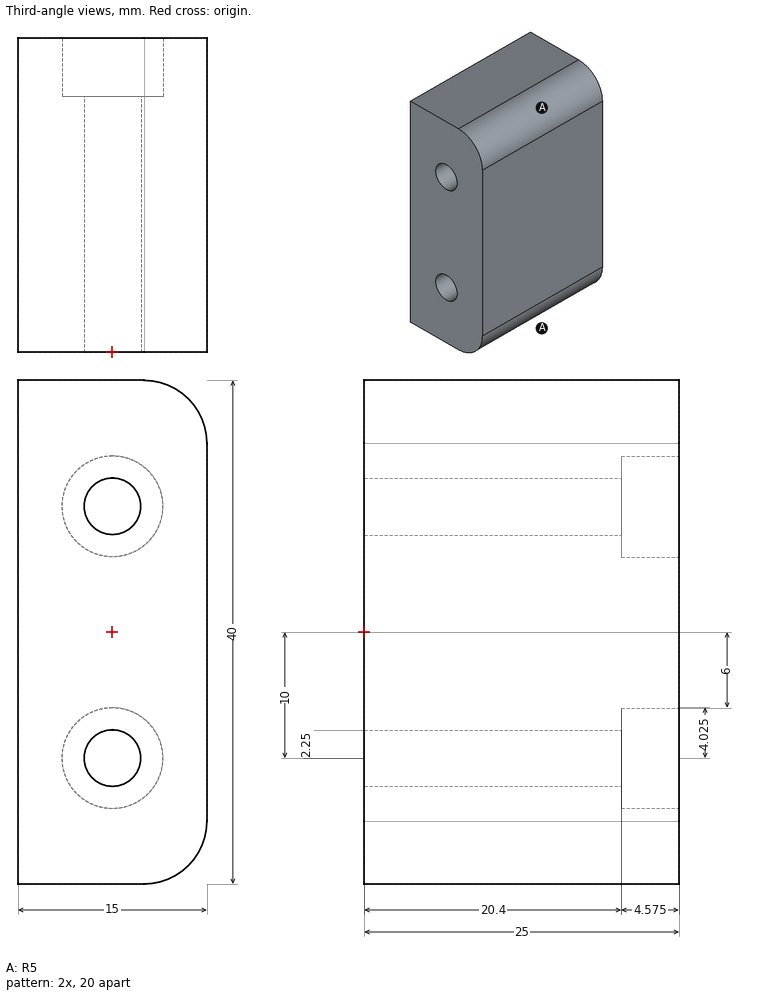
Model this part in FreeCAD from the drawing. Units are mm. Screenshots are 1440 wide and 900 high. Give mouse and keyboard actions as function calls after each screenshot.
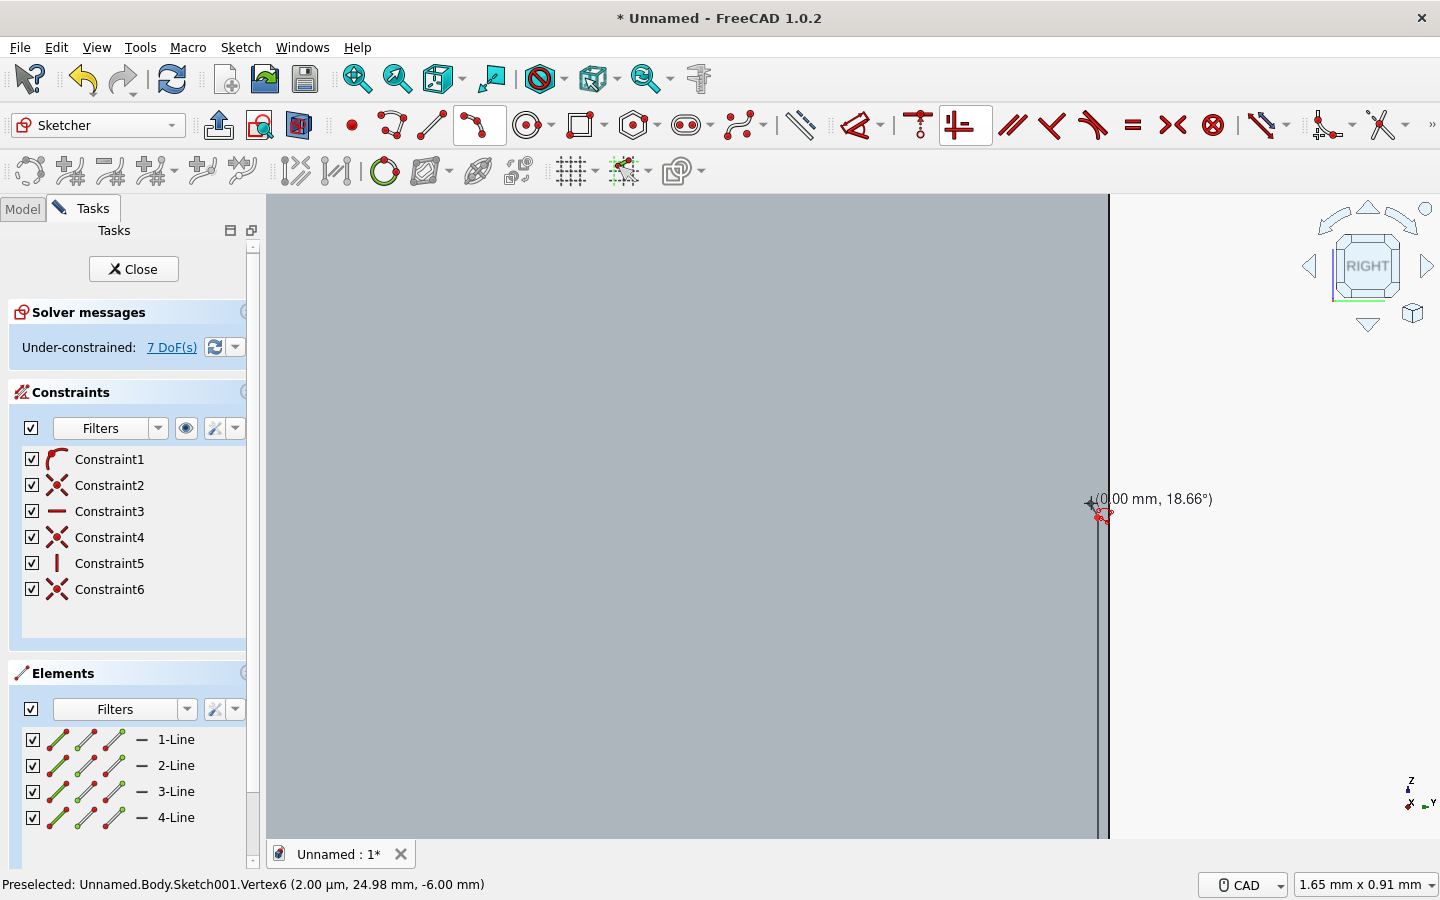
scroll(1203, 542, down, 17)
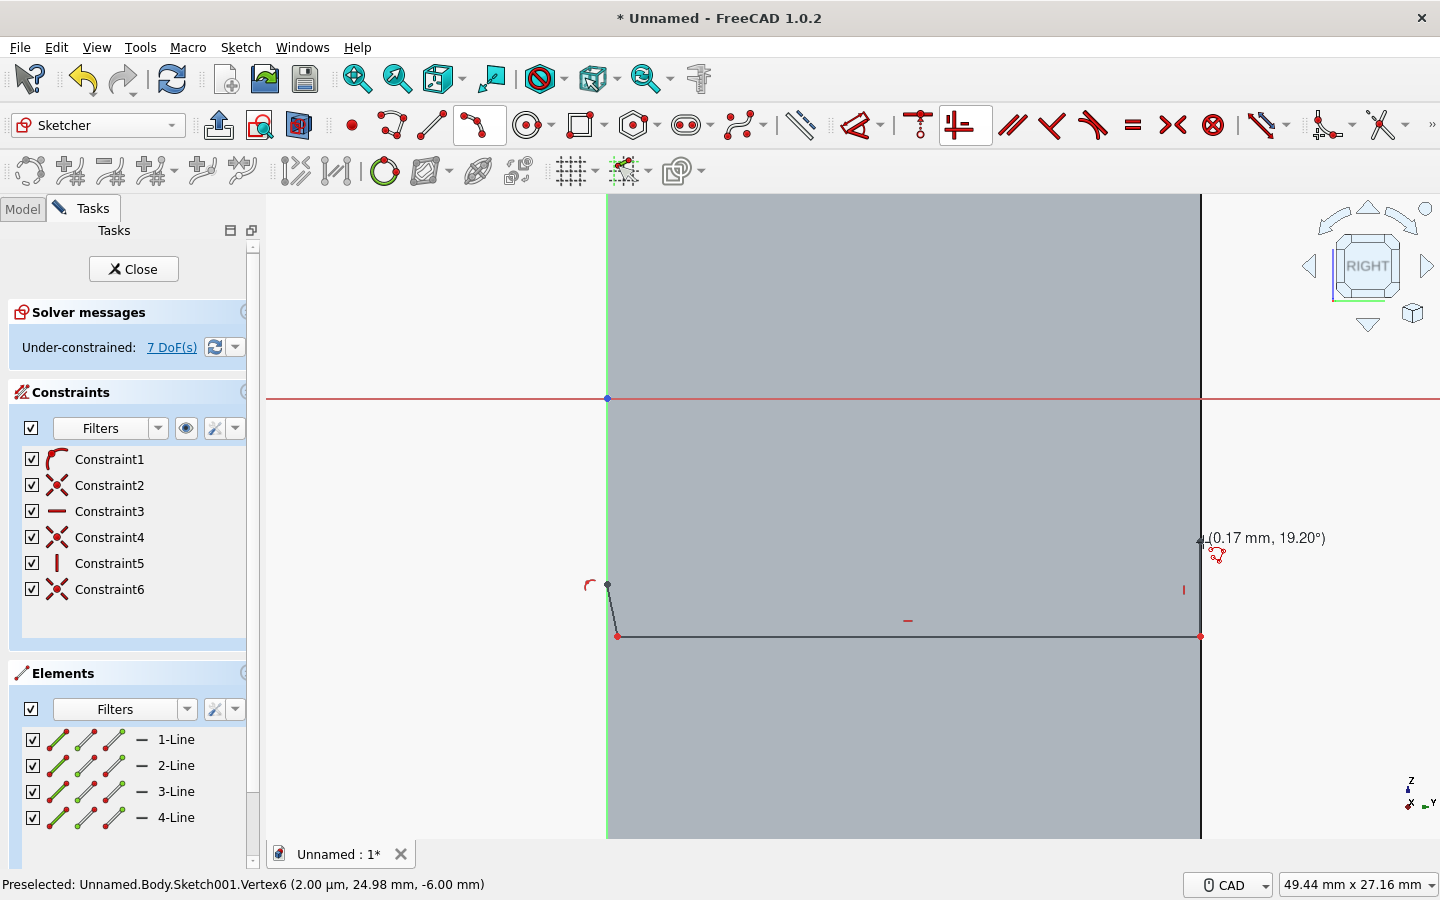
click(1091, 541)
click(1091, 583)
click(607, 584)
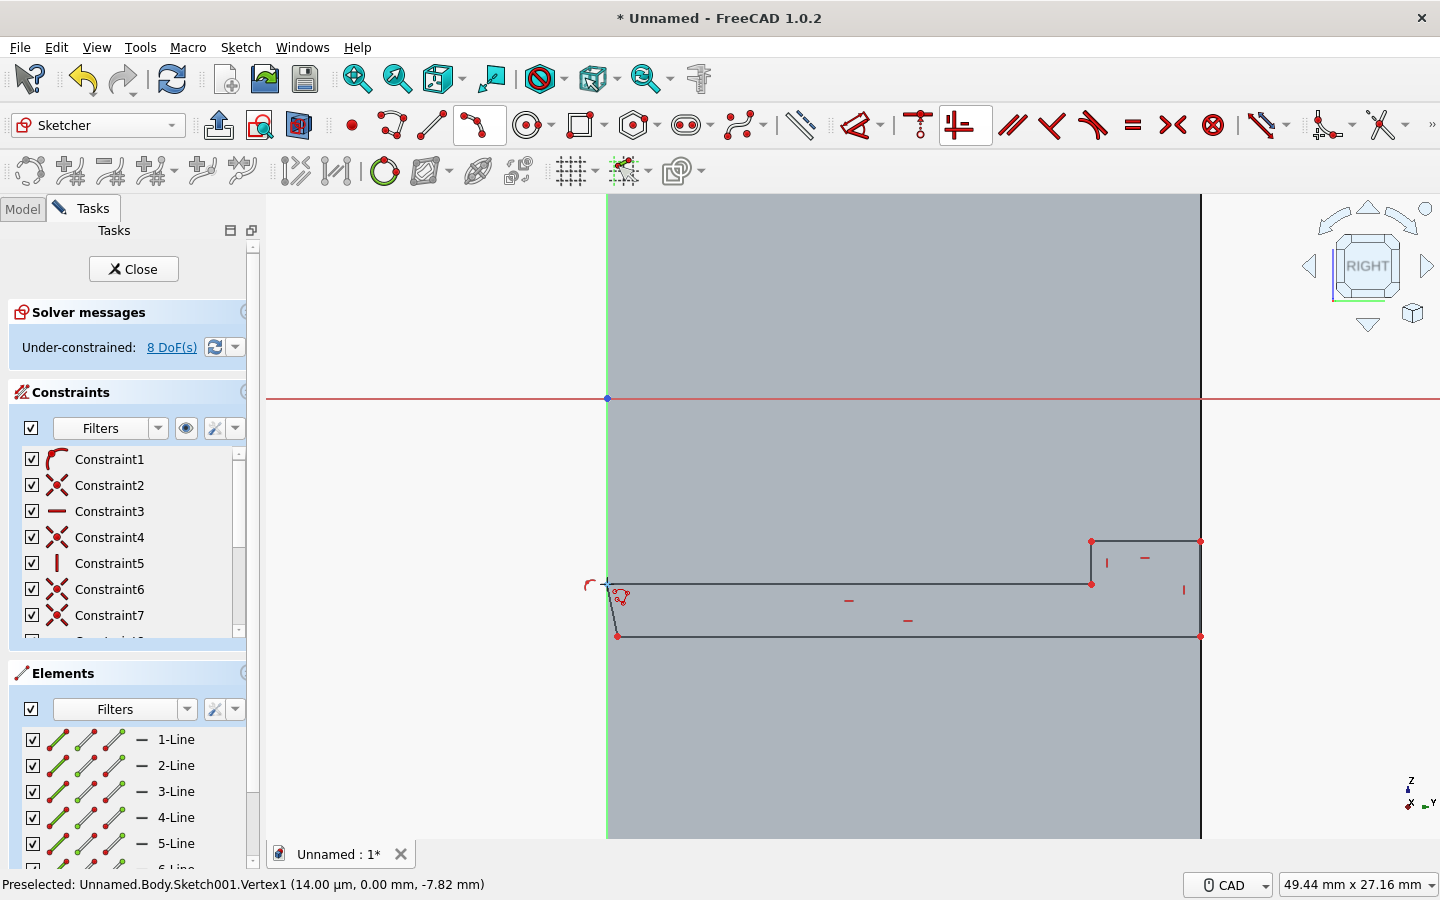
click(432, 126)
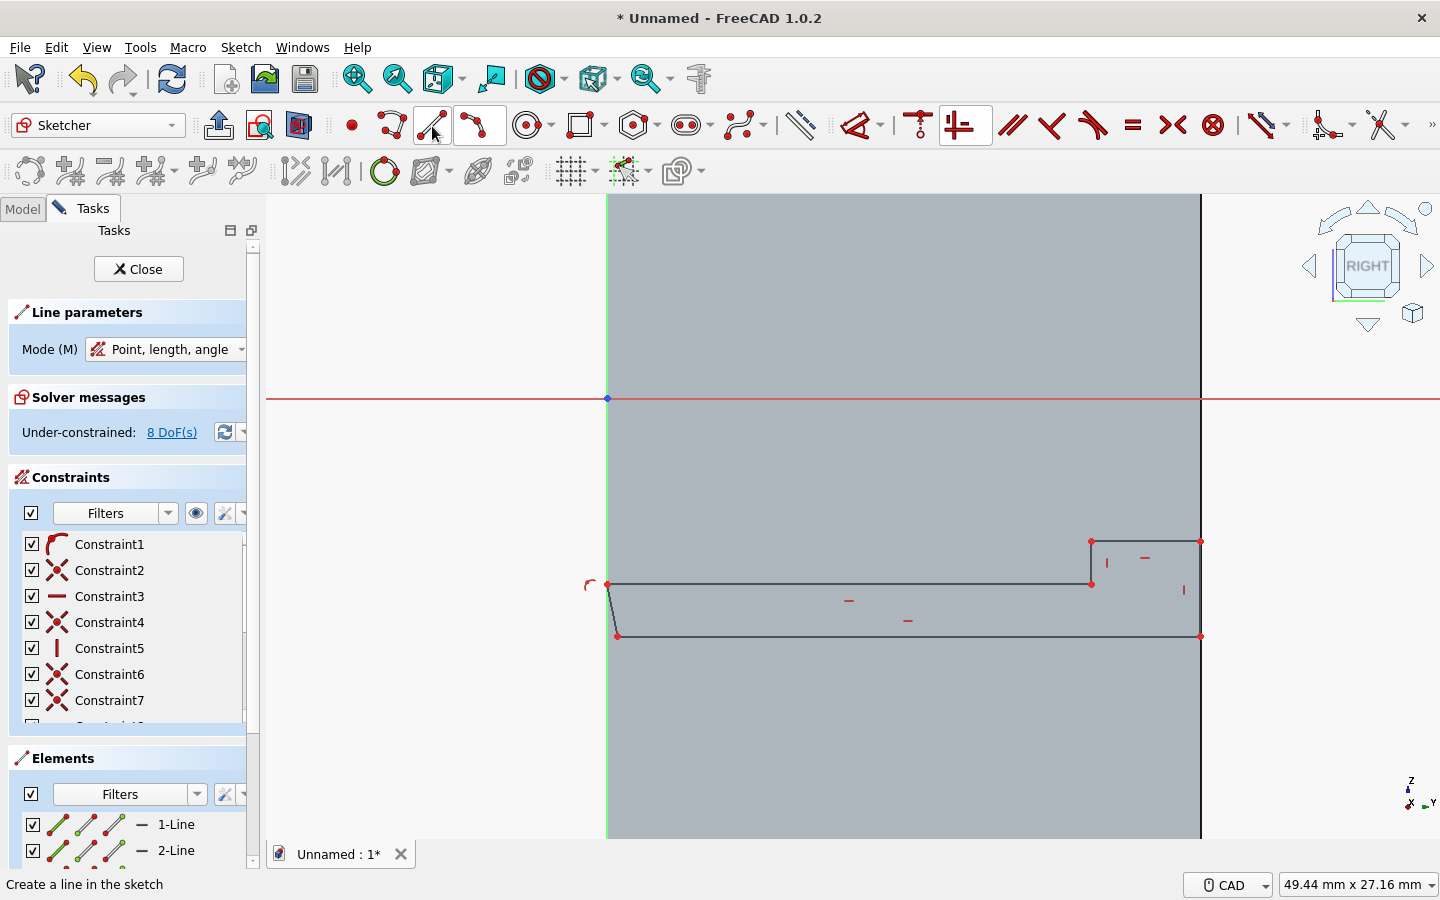
click(548, 636)
click(370, 636)
key(Escape)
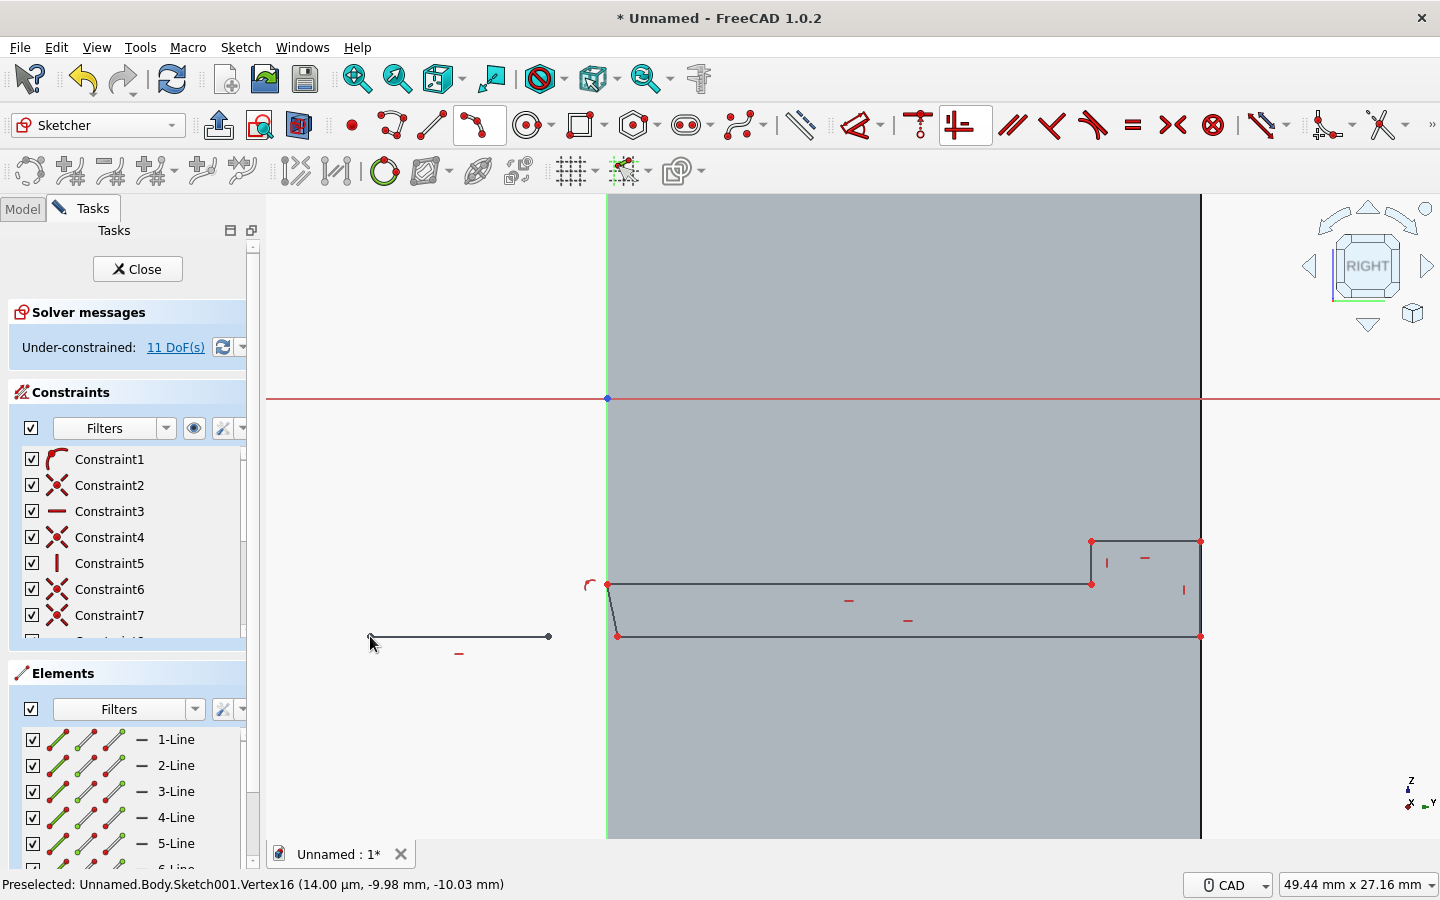
click(495, 637)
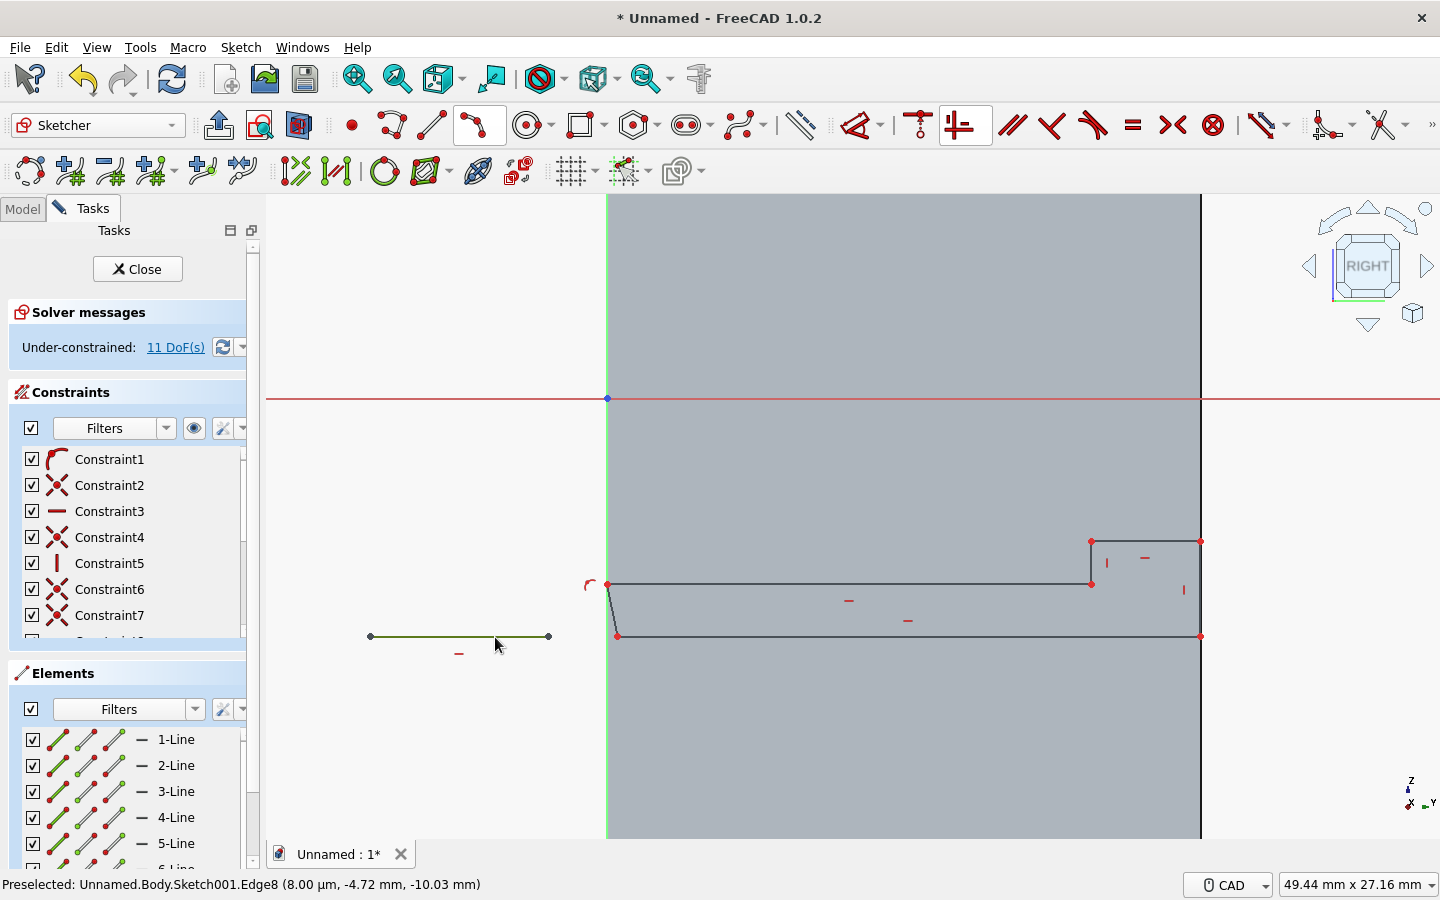
click(802, 126)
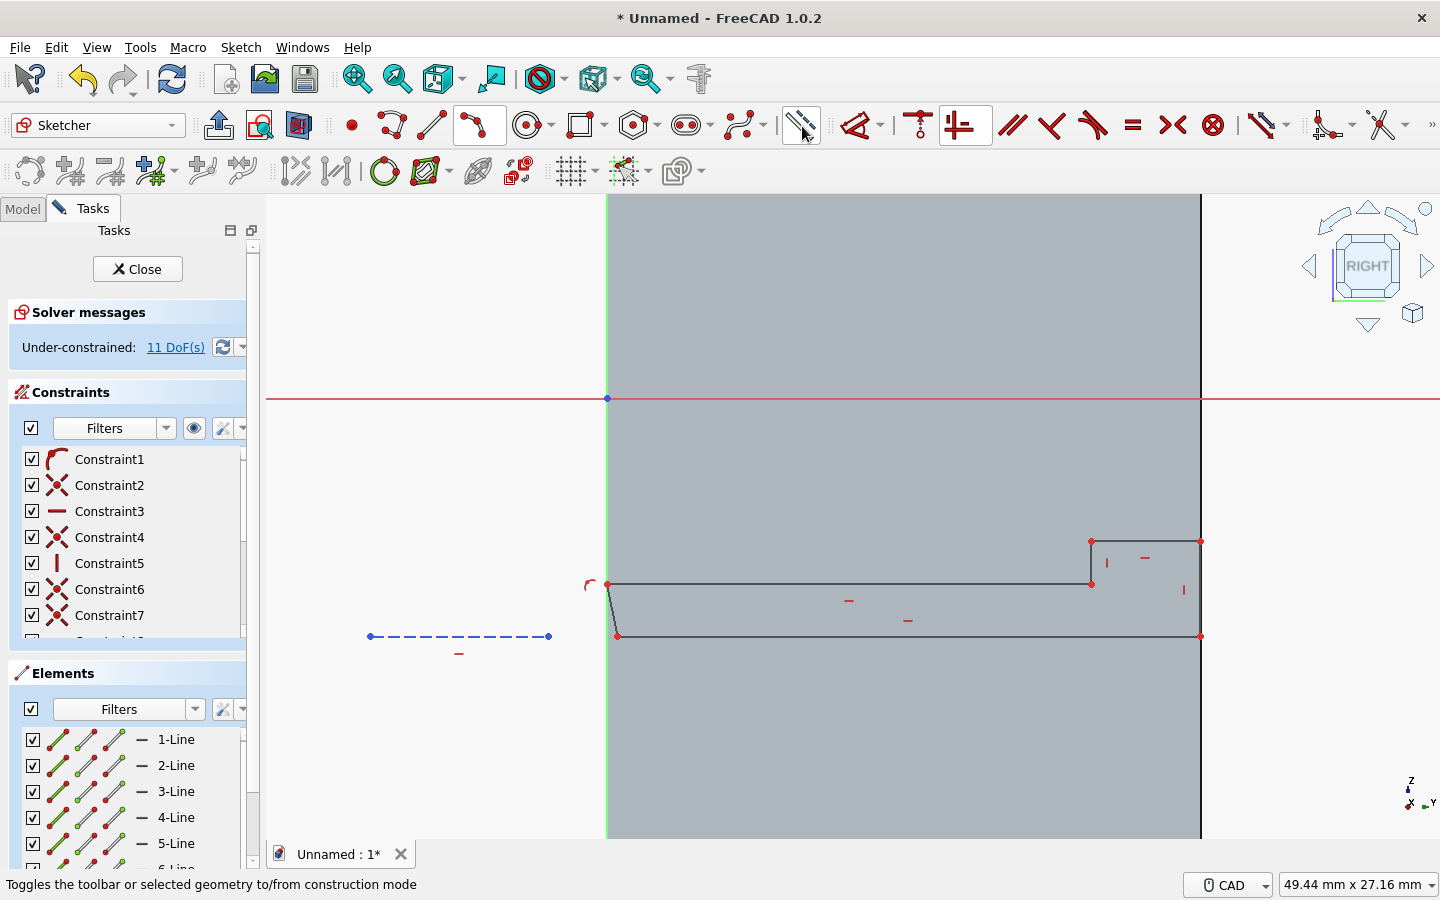
click(610, 600)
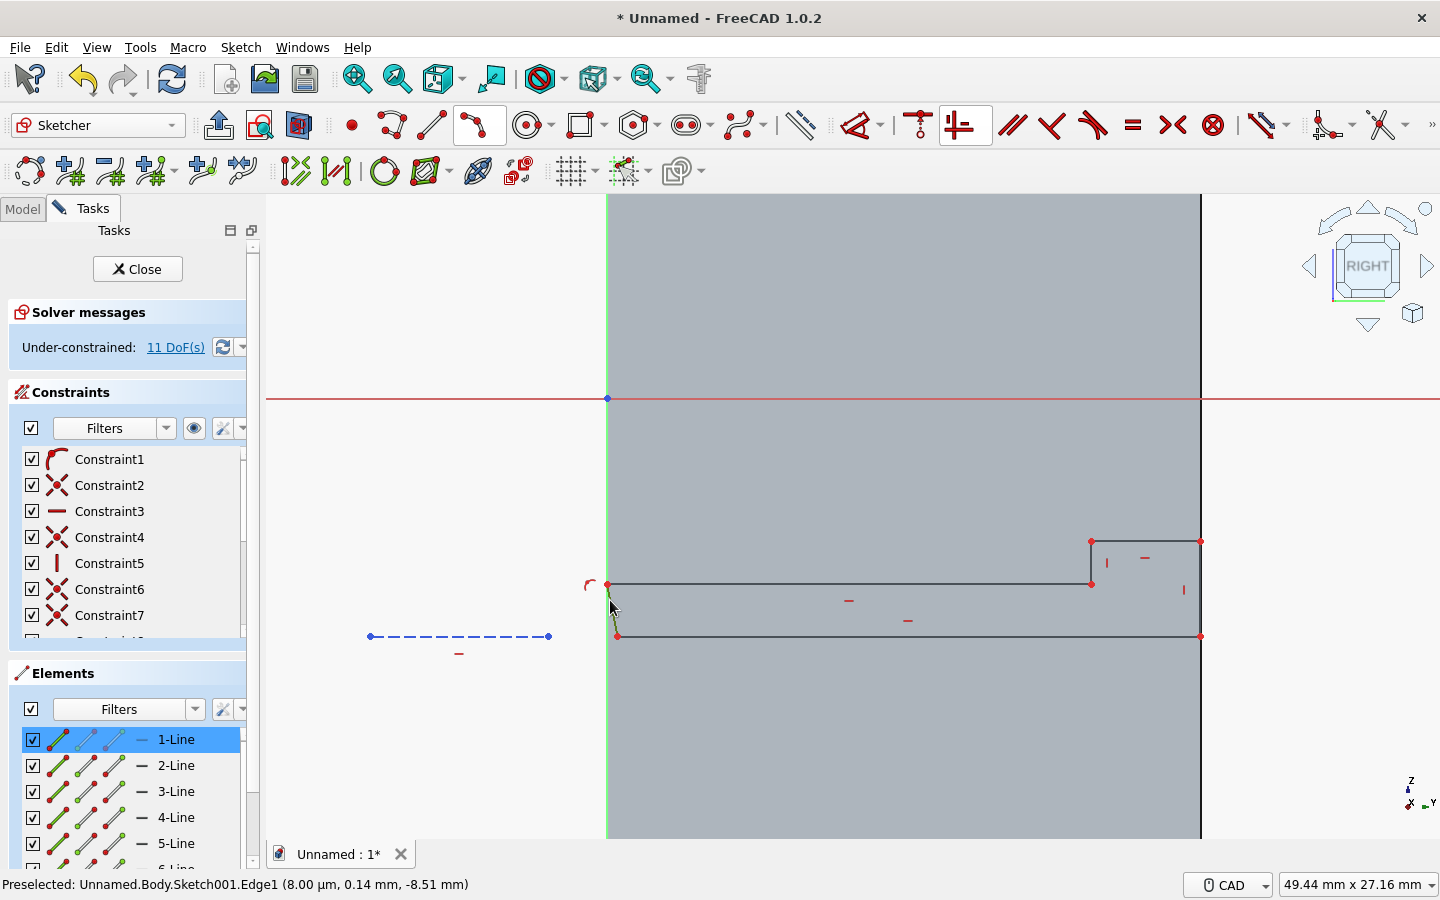
key(v)